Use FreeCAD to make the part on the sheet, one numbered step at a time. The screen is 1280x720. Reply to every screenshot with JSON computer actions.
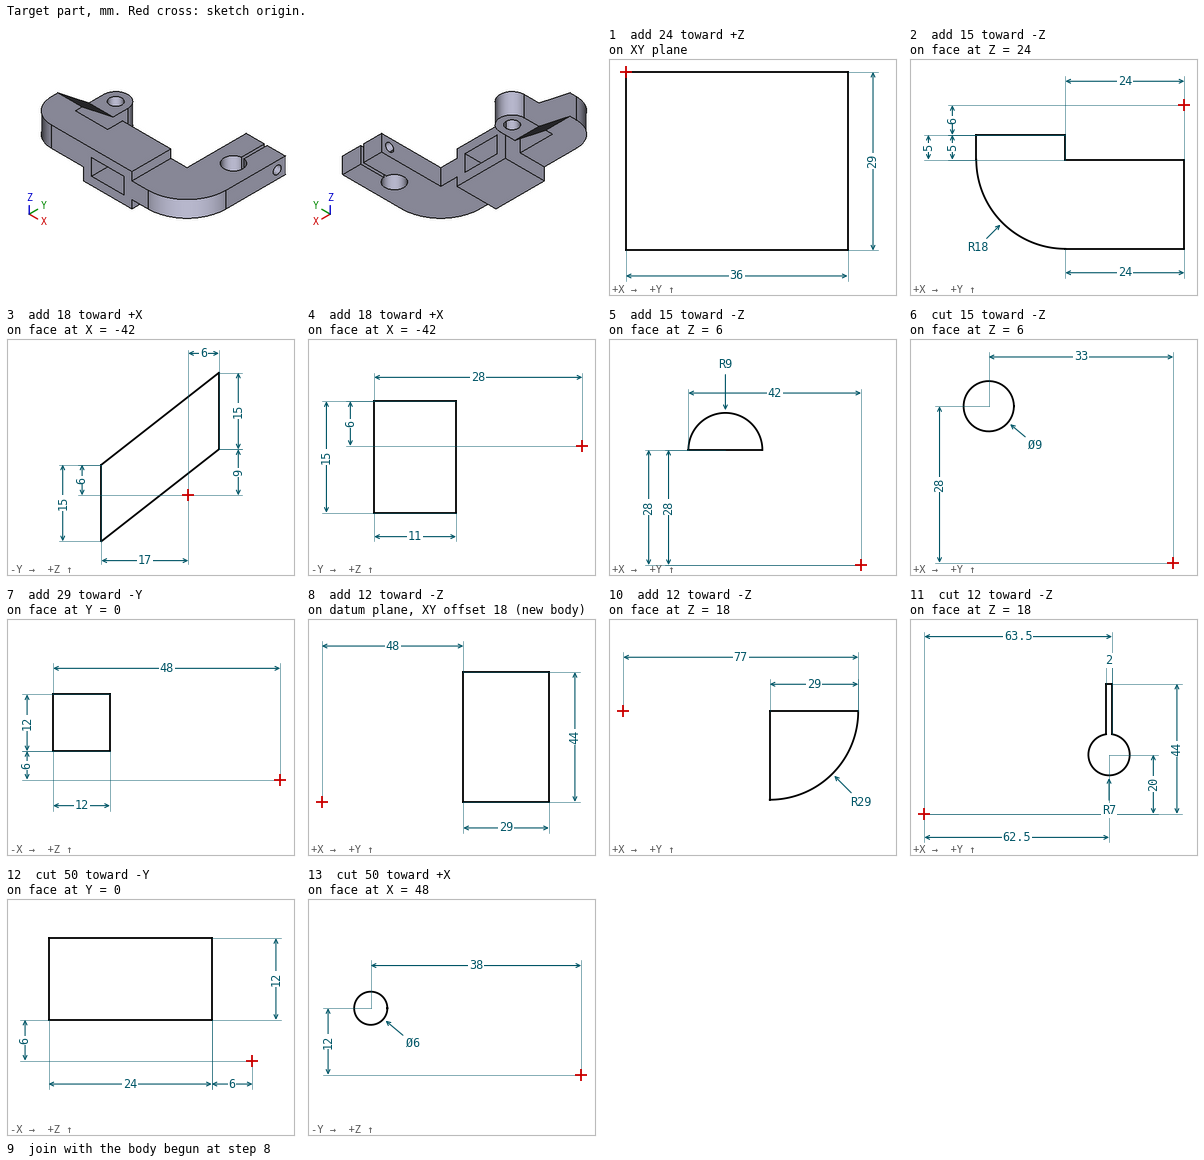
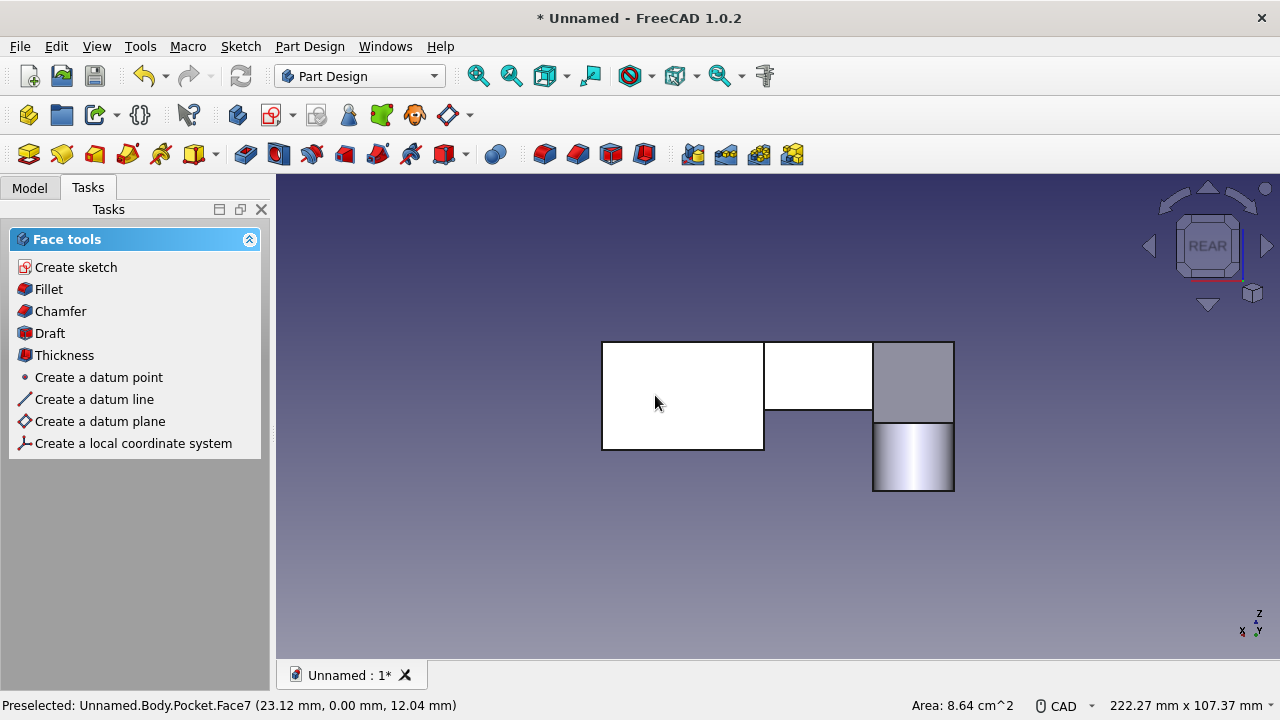
{"action": "left_click", "coordinate": [270, 116]}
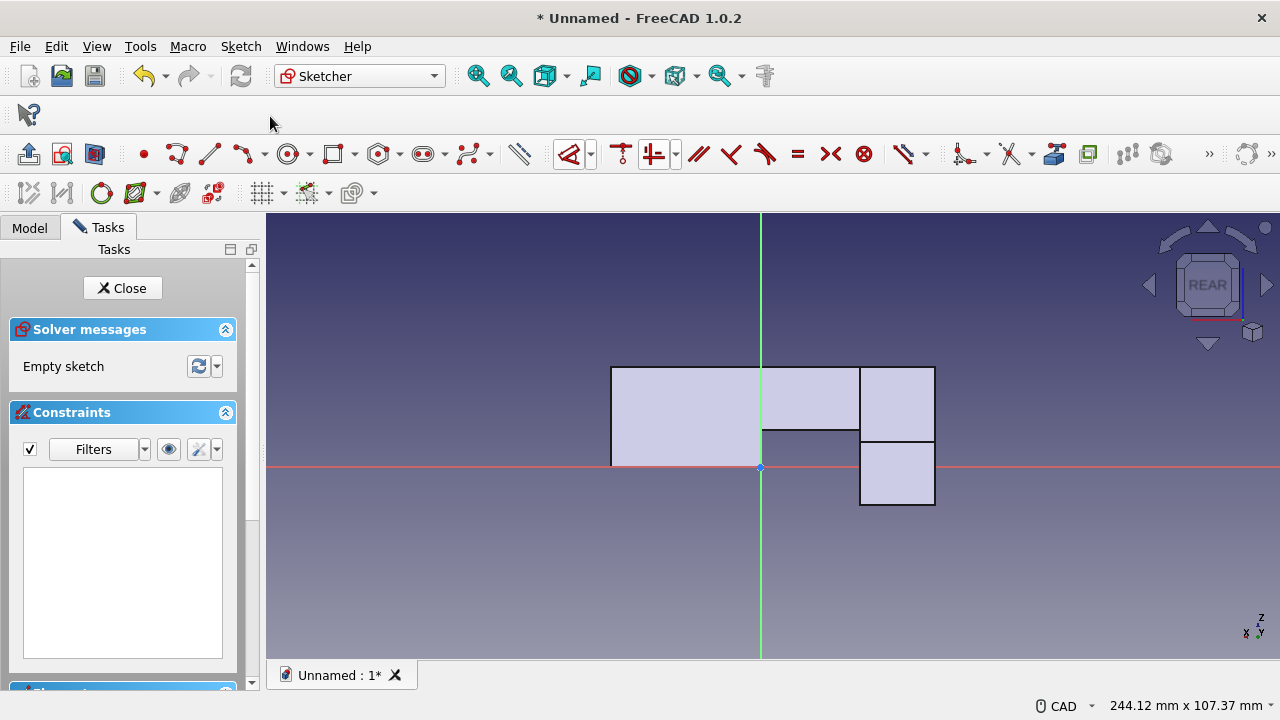
{"action": "scroll", "coordinate": [563, 414], "scroll_direction": "up", "scroll_amount": 9}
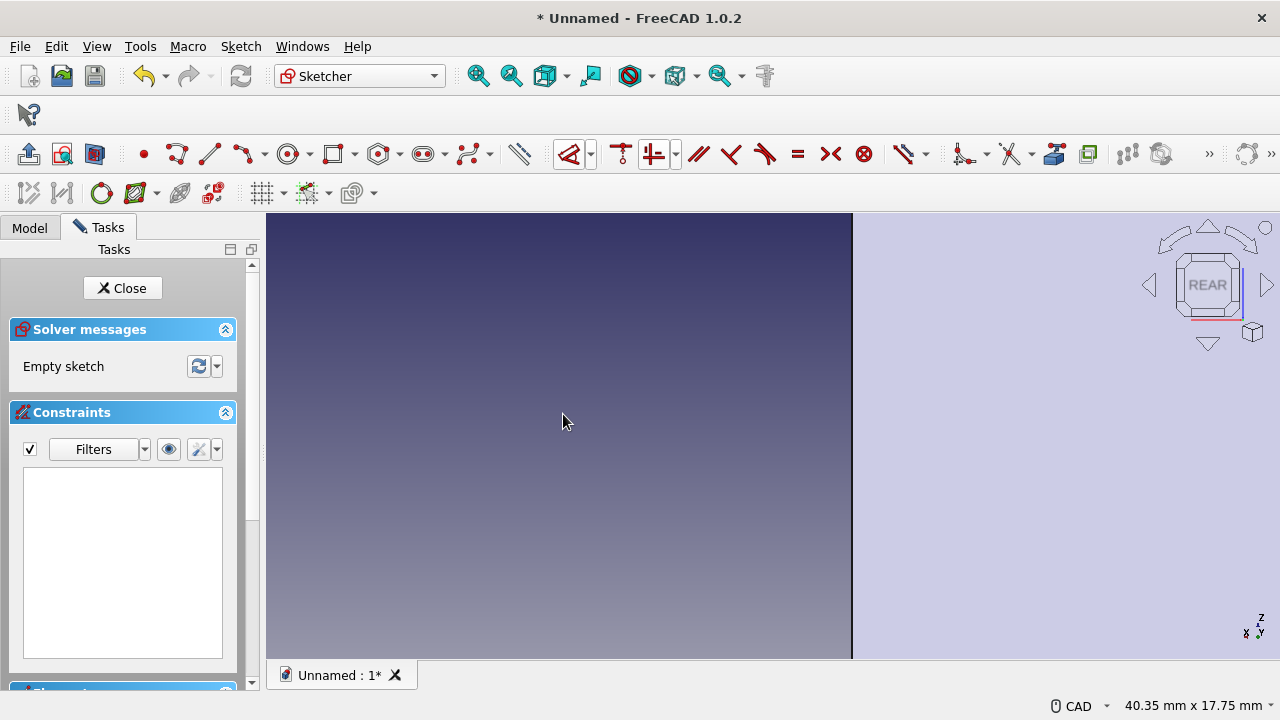
{"action": "left_click", "coordinate": [332, 154]}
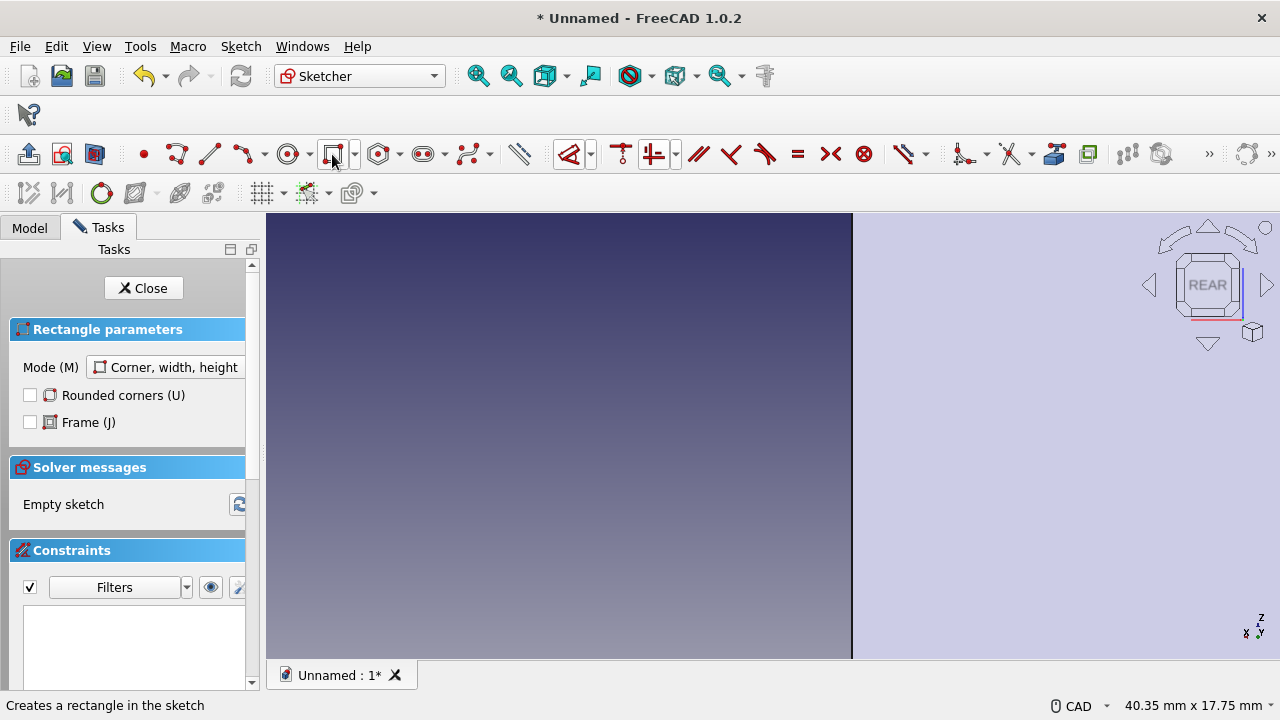
{"action": "left_click", "coordinate": [550, 281]}
{"action": "mouse_move", "coordinate": [852, 583]}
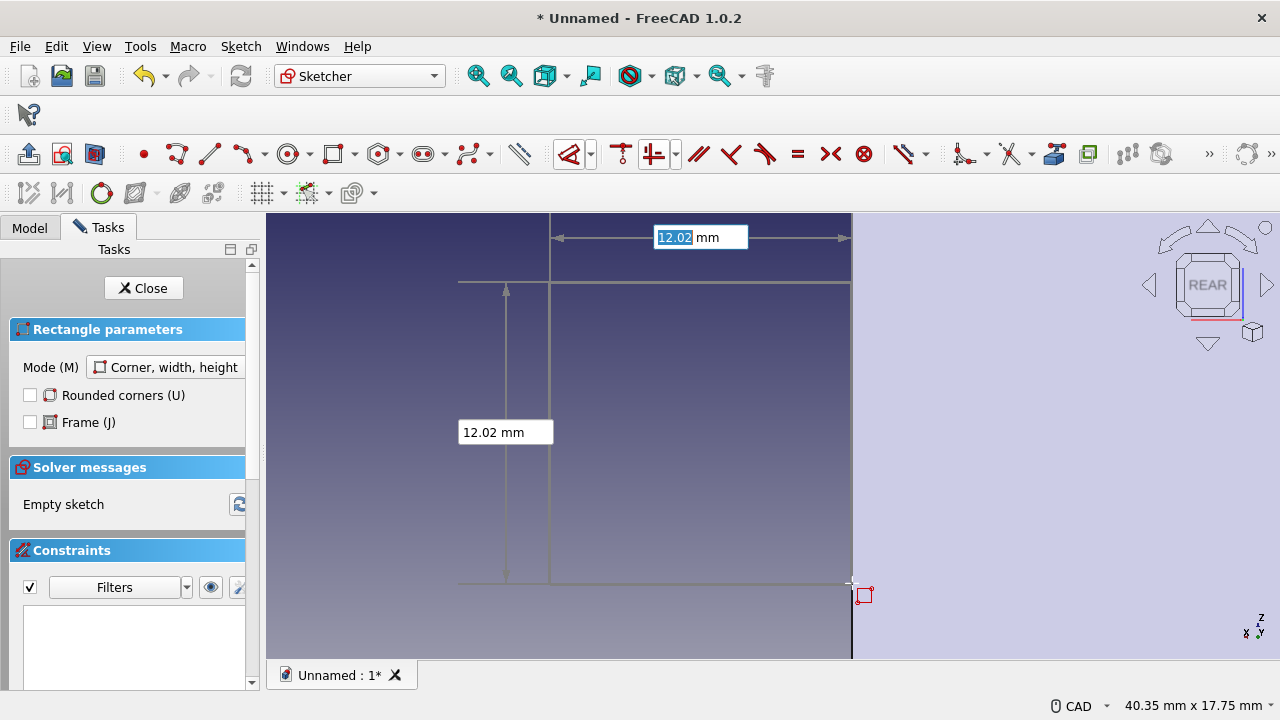
{"action": "type", "text": "12"}
{"action": "key", "text": "Tab"}
{"action": "type", "text": "12"}
{"action": "key", "text": "Return"}
{"action": "key", "text": "Escape"}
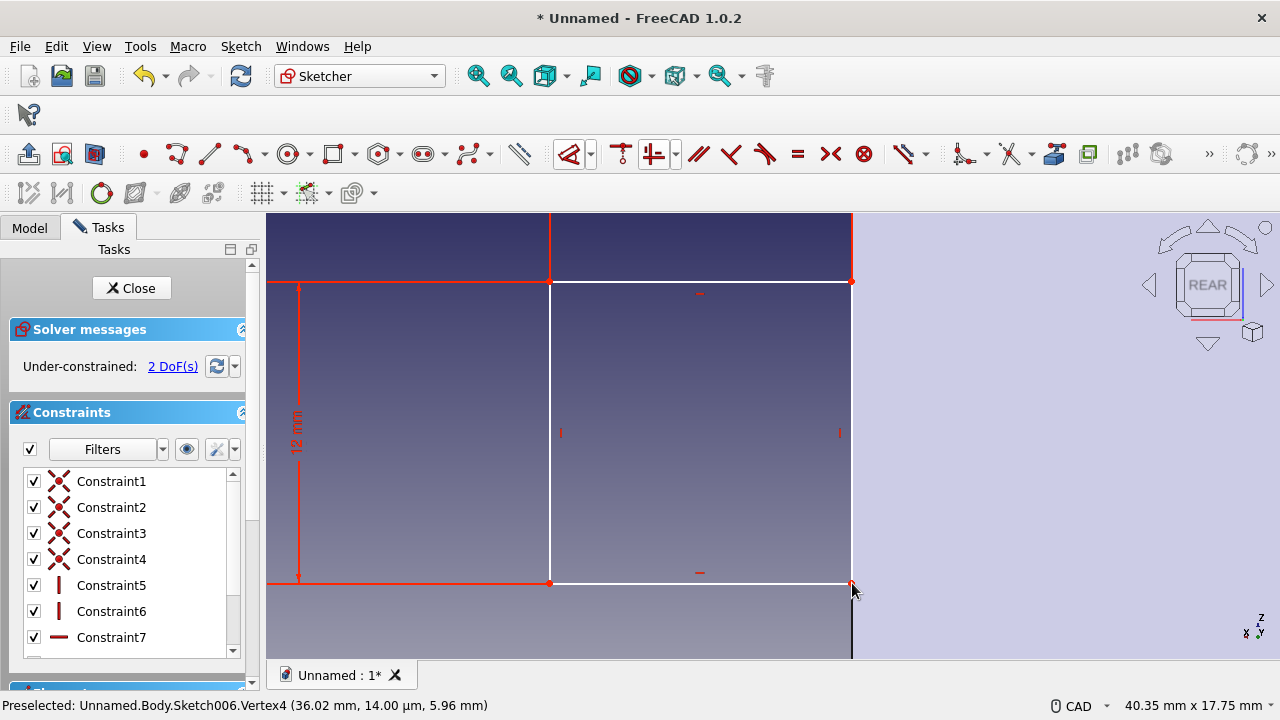
{"action": "left_click", "coordinate": [550, 584]}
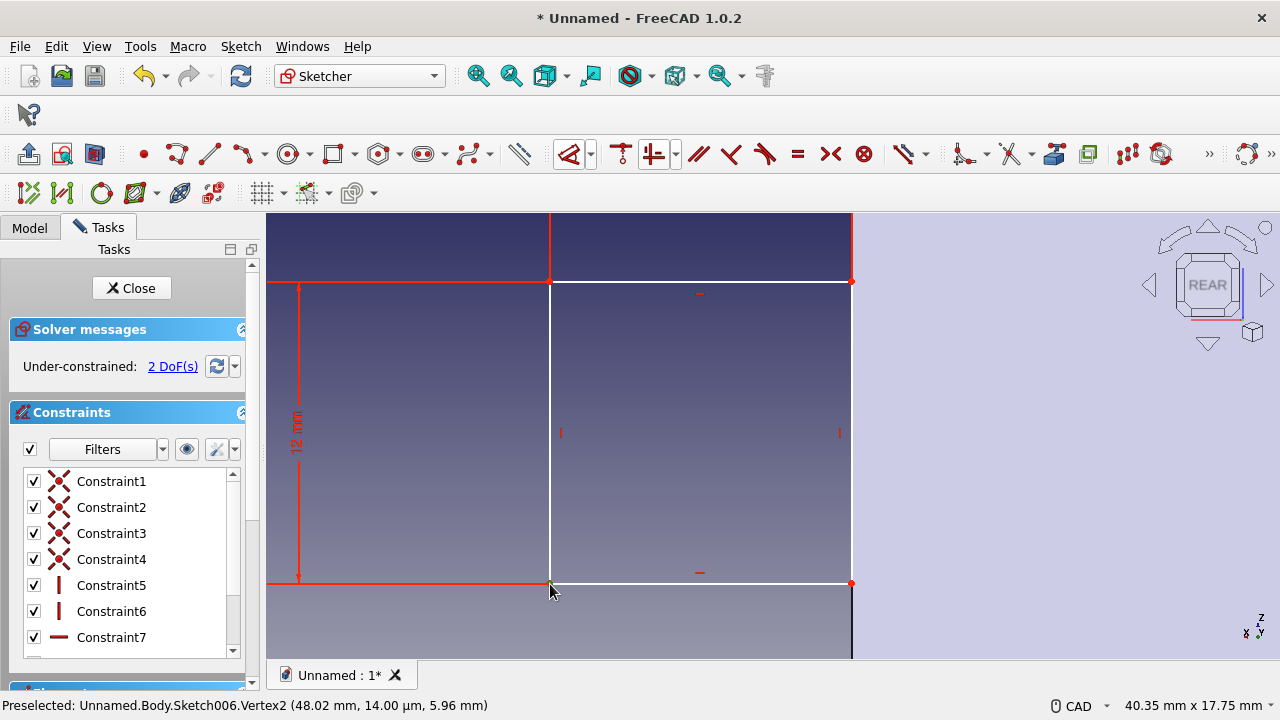
{"action": "key", "text": "i"}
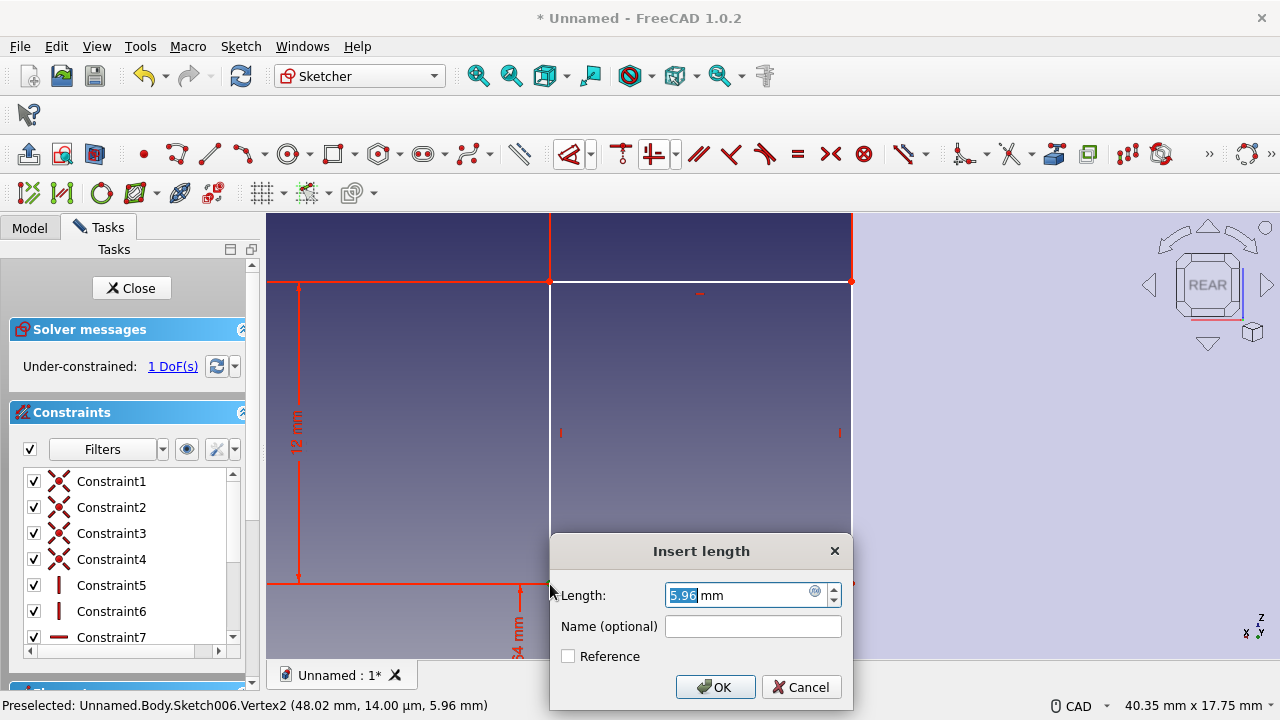
{"action": "type", "text": "6"}
{"action": "key", "text": "Return"}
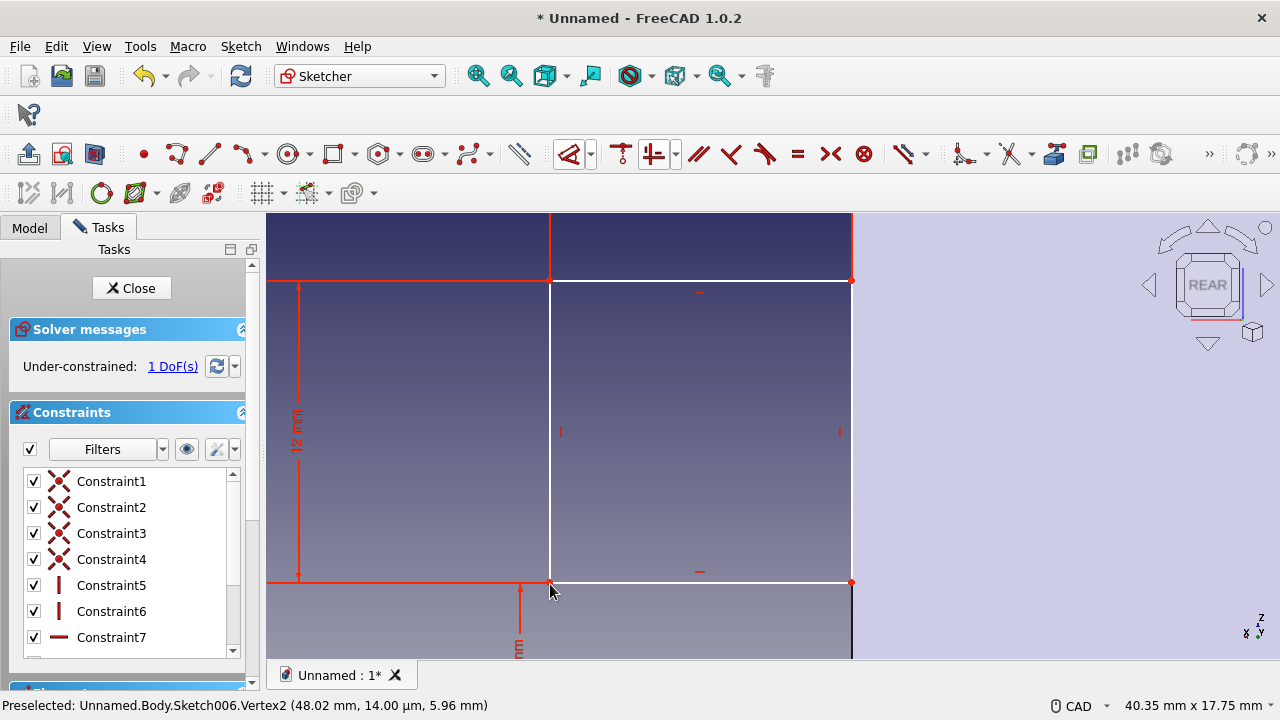
{"action": "left_click", "coordinate": [550, 281]}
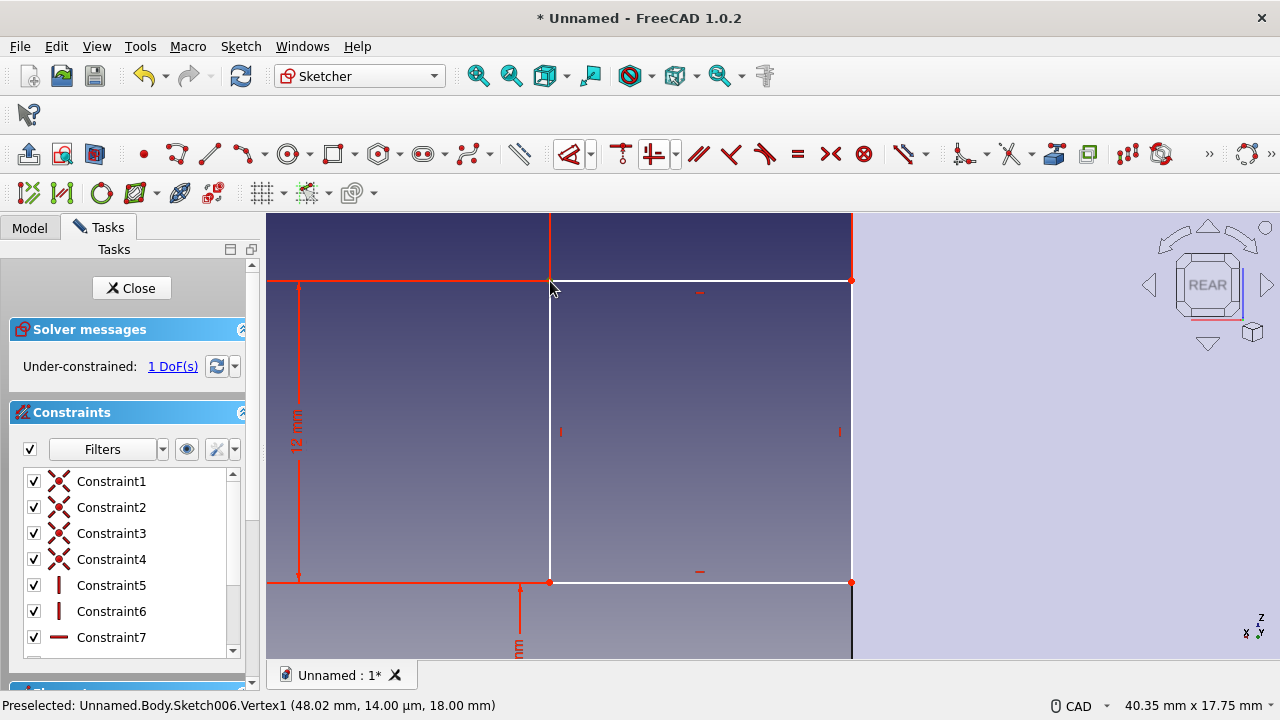
{"action": "left_click", "coordinate": [590, 154]}